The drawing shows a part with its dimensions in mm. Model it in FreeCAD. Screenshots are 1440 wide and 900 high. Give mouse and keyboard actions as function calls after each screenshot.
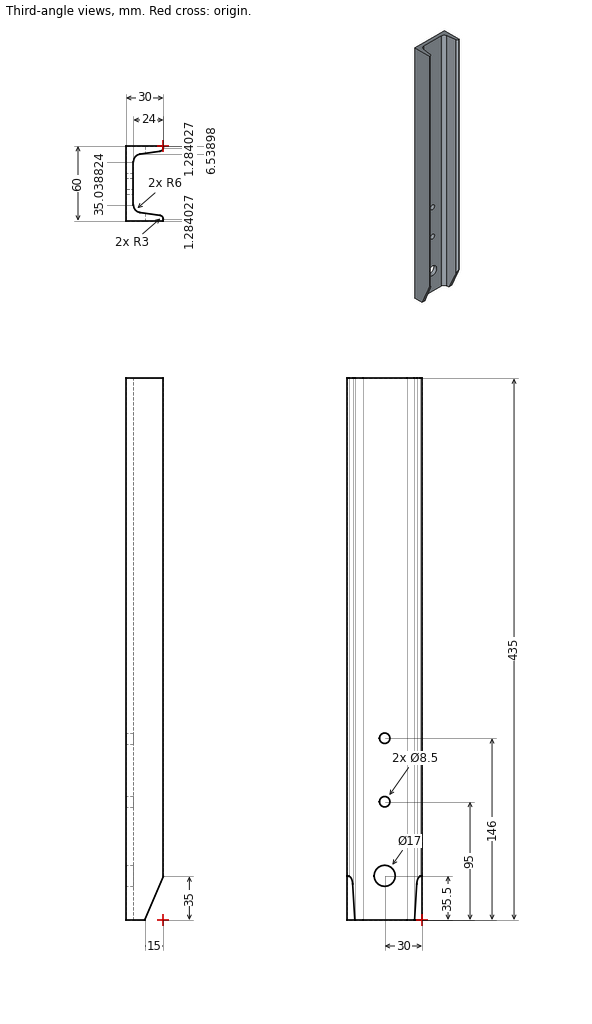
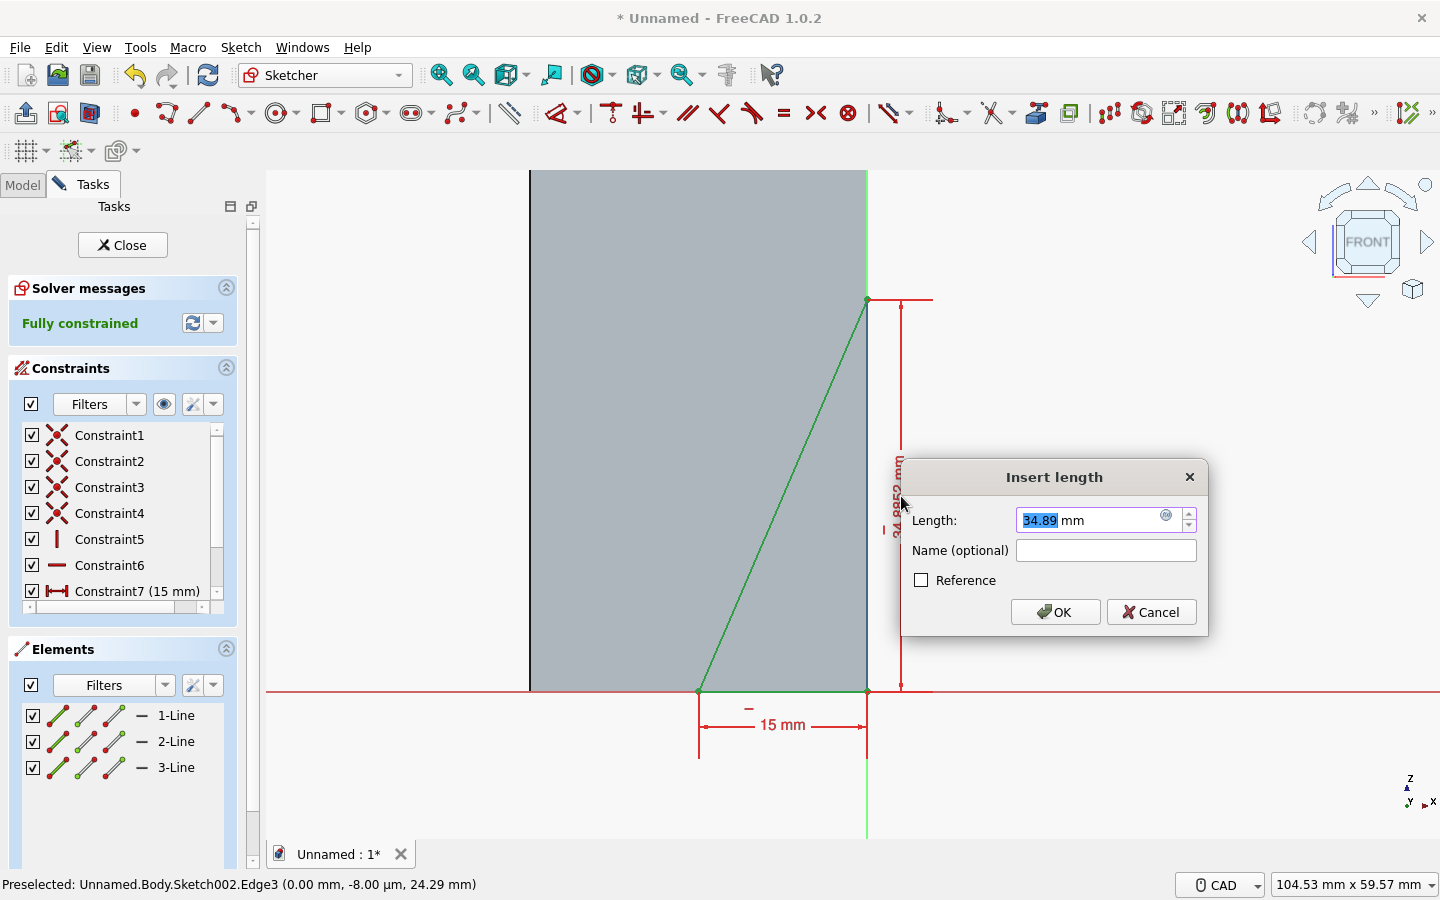
text(35)
key(Return)
key(Escape)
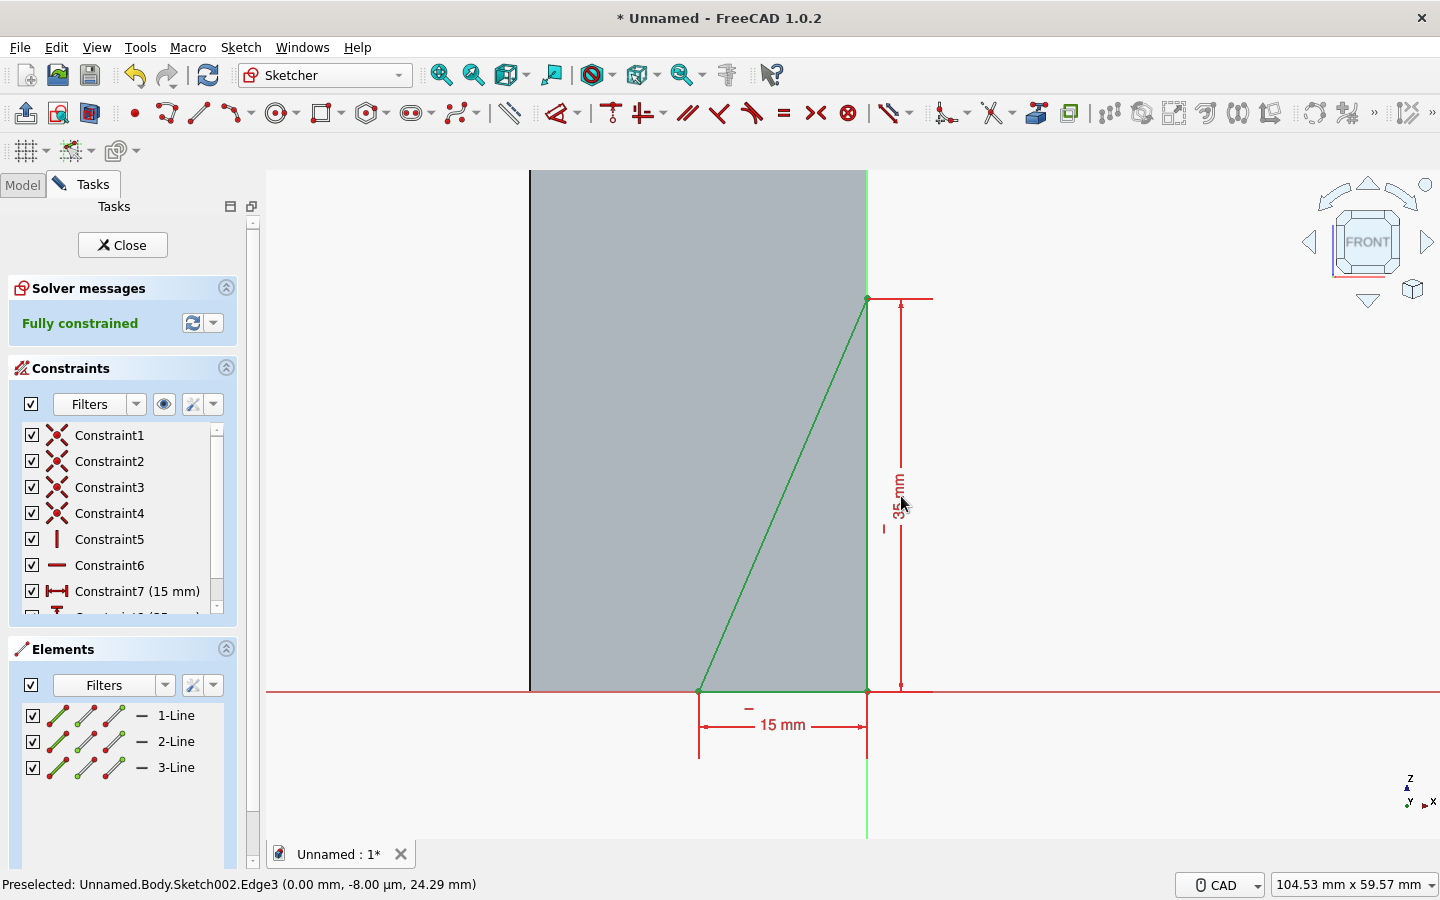
click(123, 245)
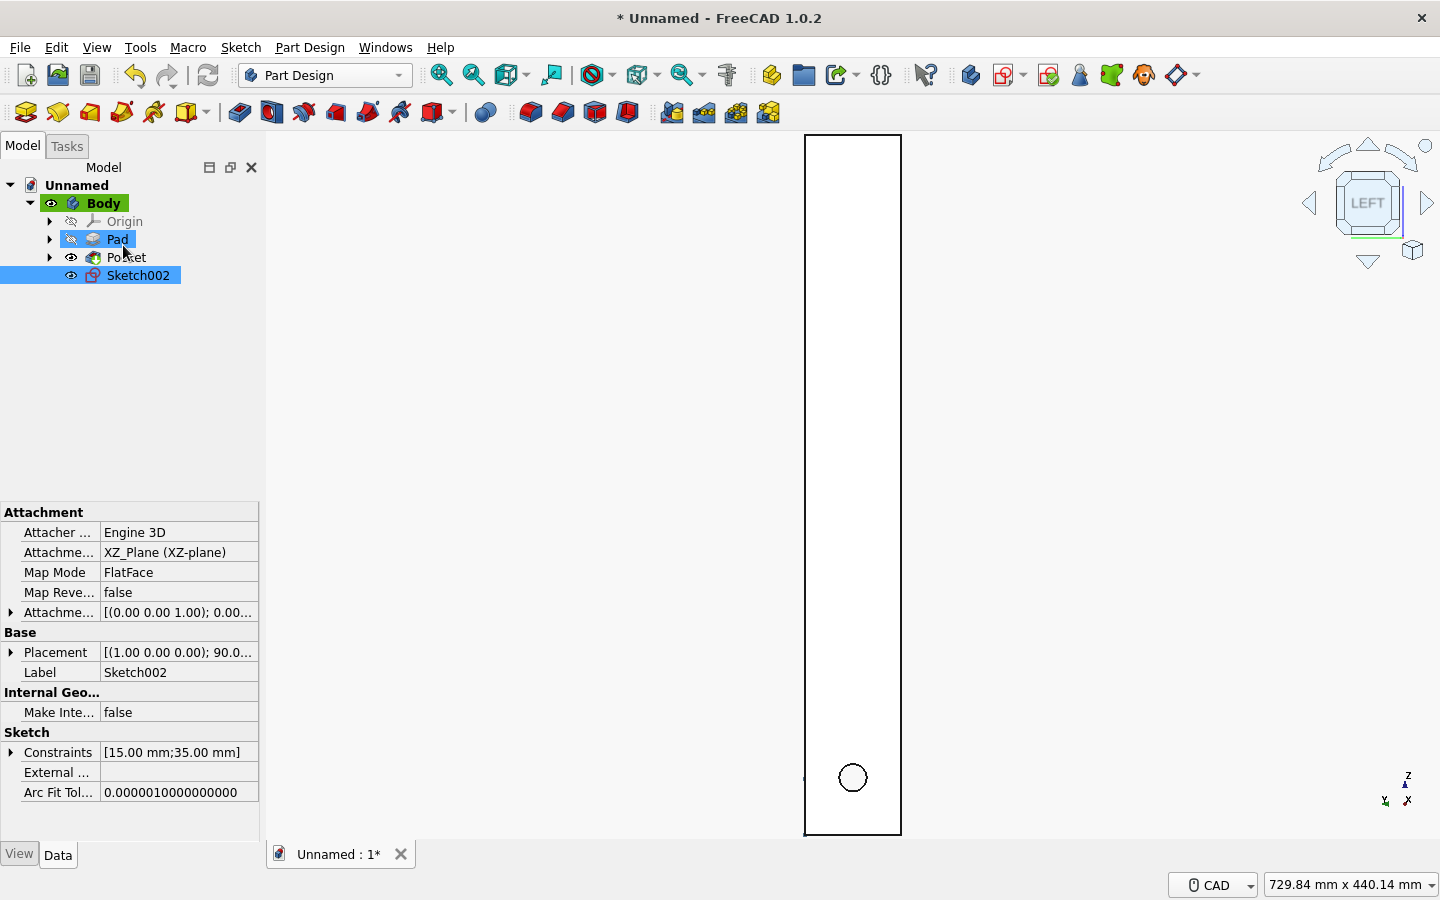
click(240, 112)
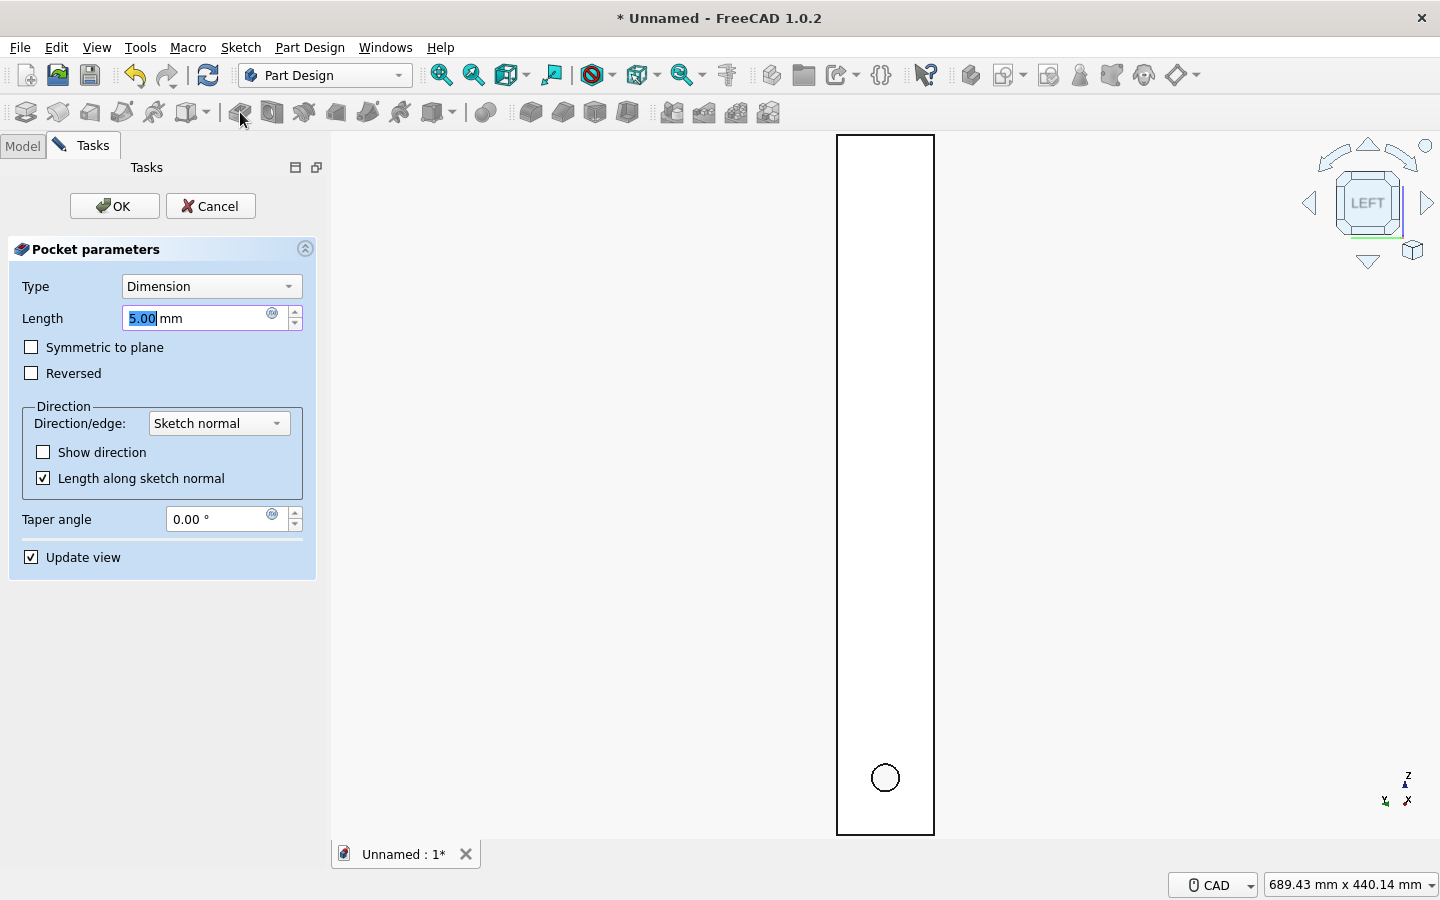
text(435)
key(Tab)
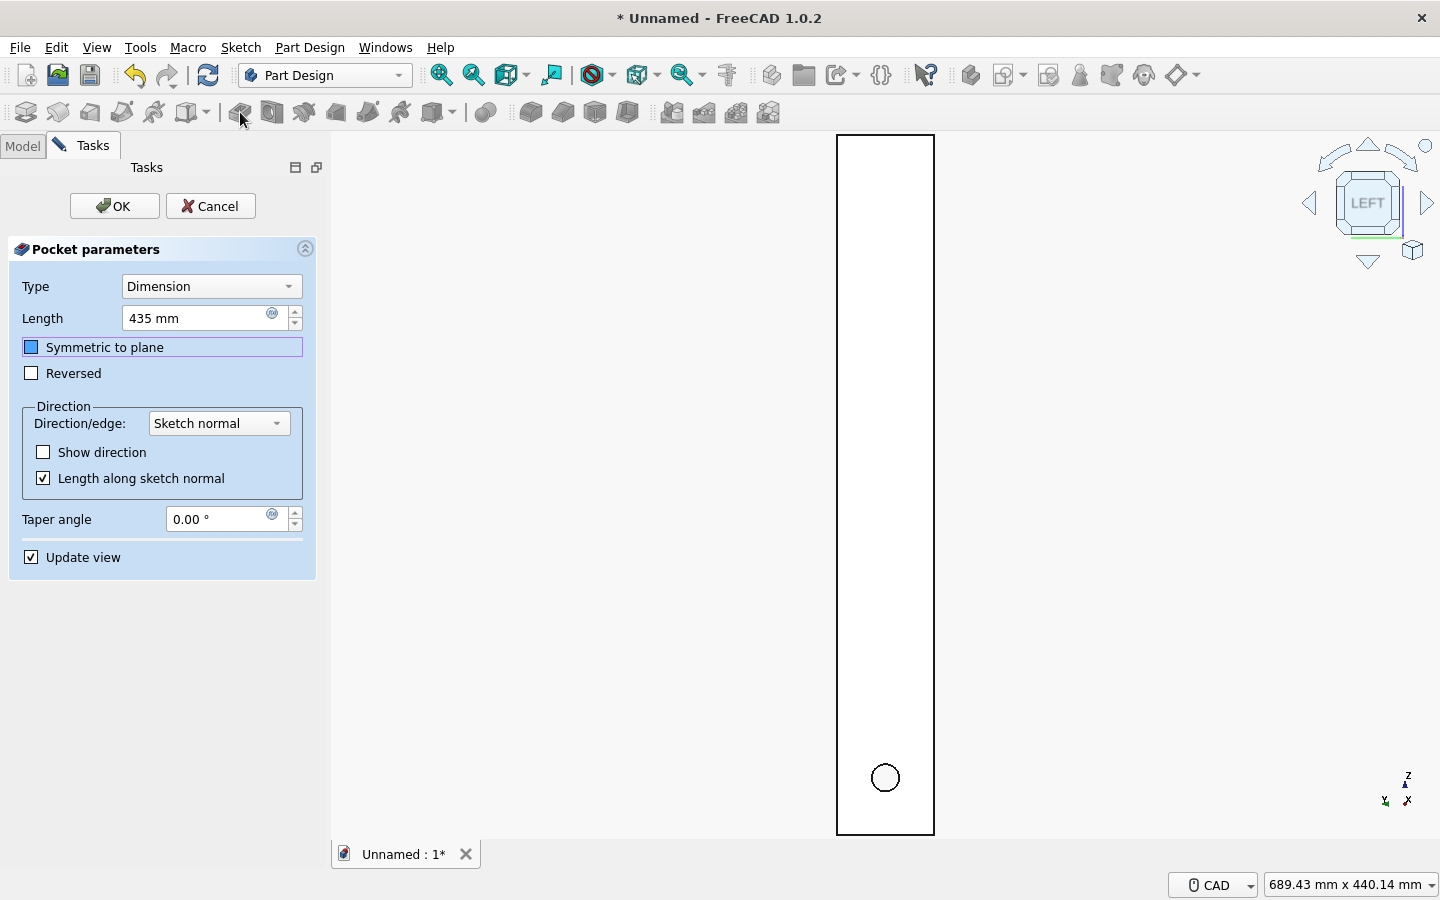
click(30, 373)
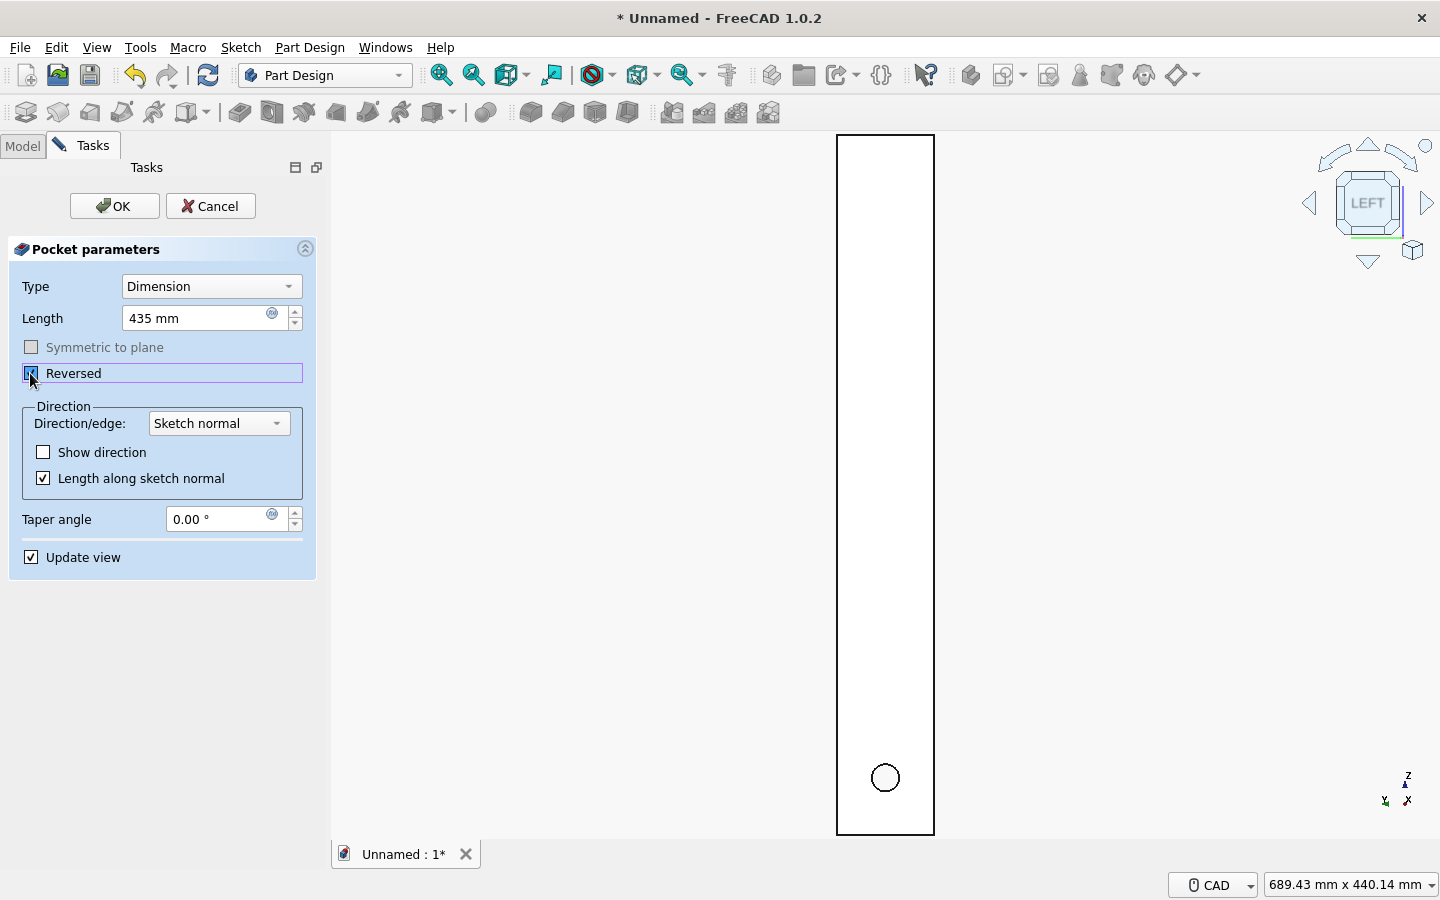
click(115, 206)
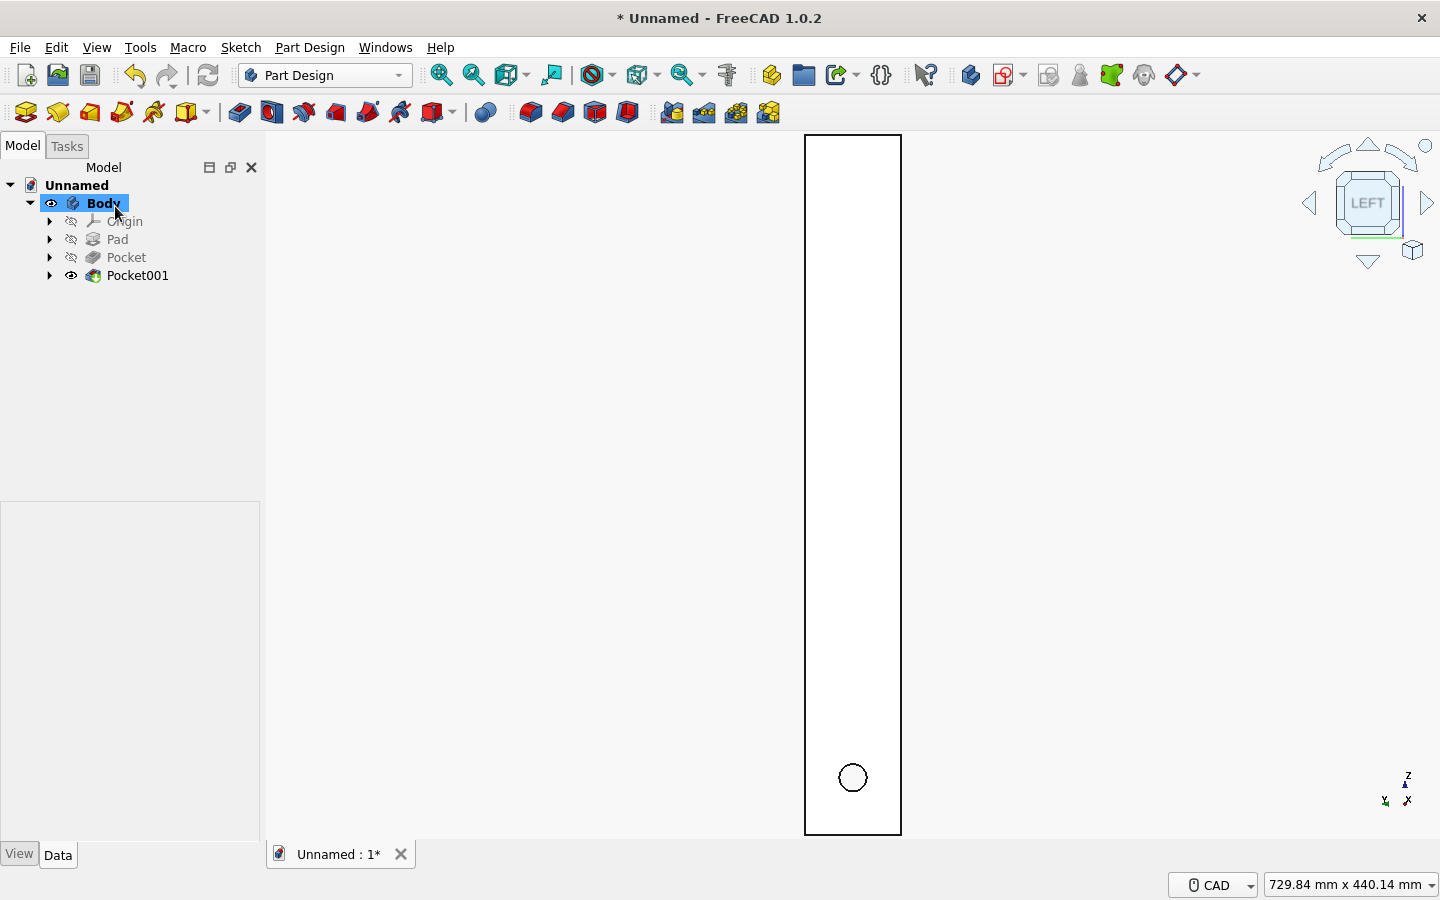
click(853, 184)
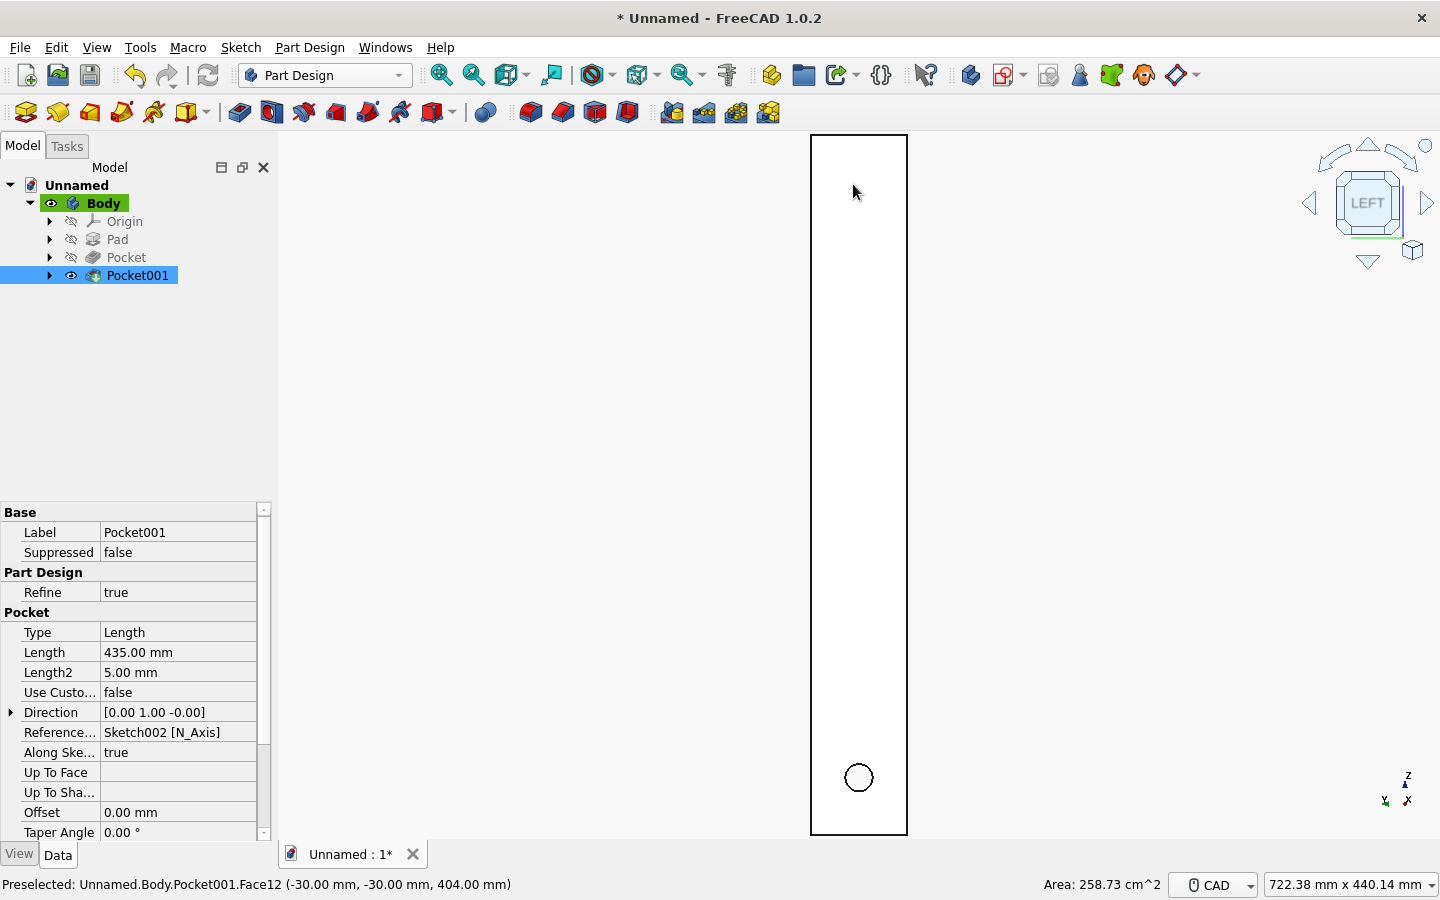
click(1004, 76)